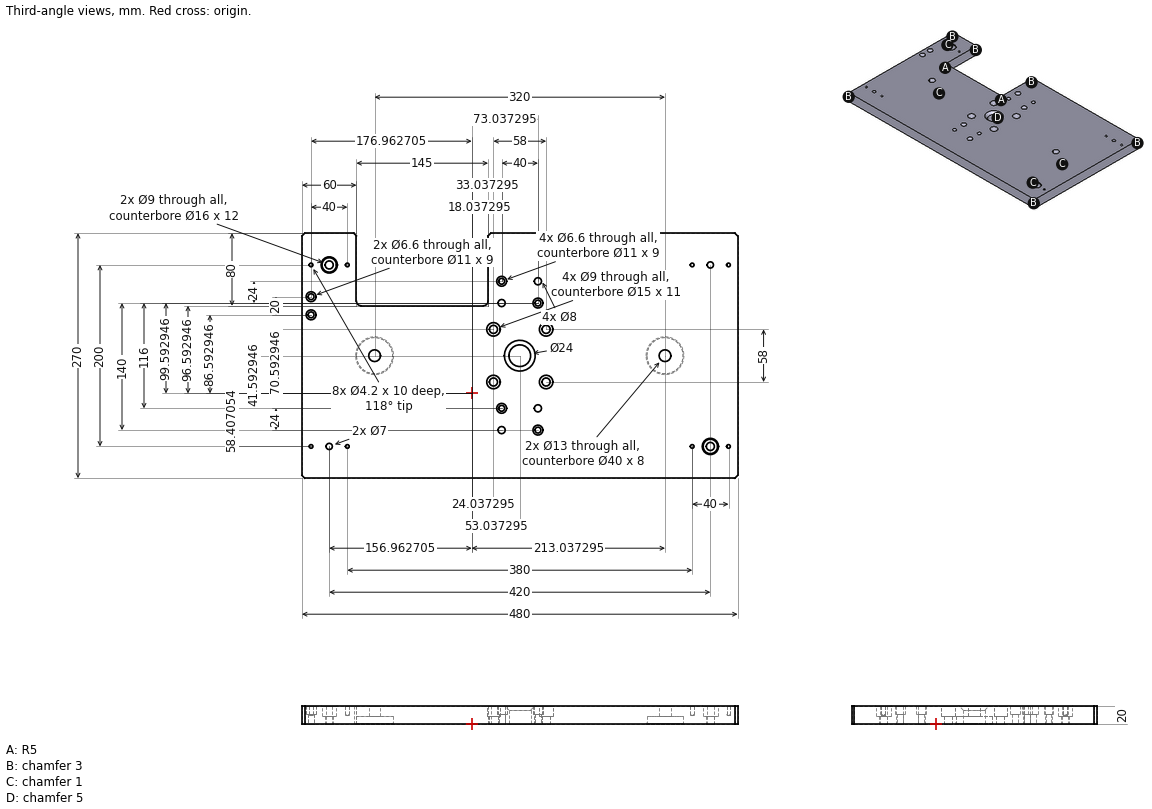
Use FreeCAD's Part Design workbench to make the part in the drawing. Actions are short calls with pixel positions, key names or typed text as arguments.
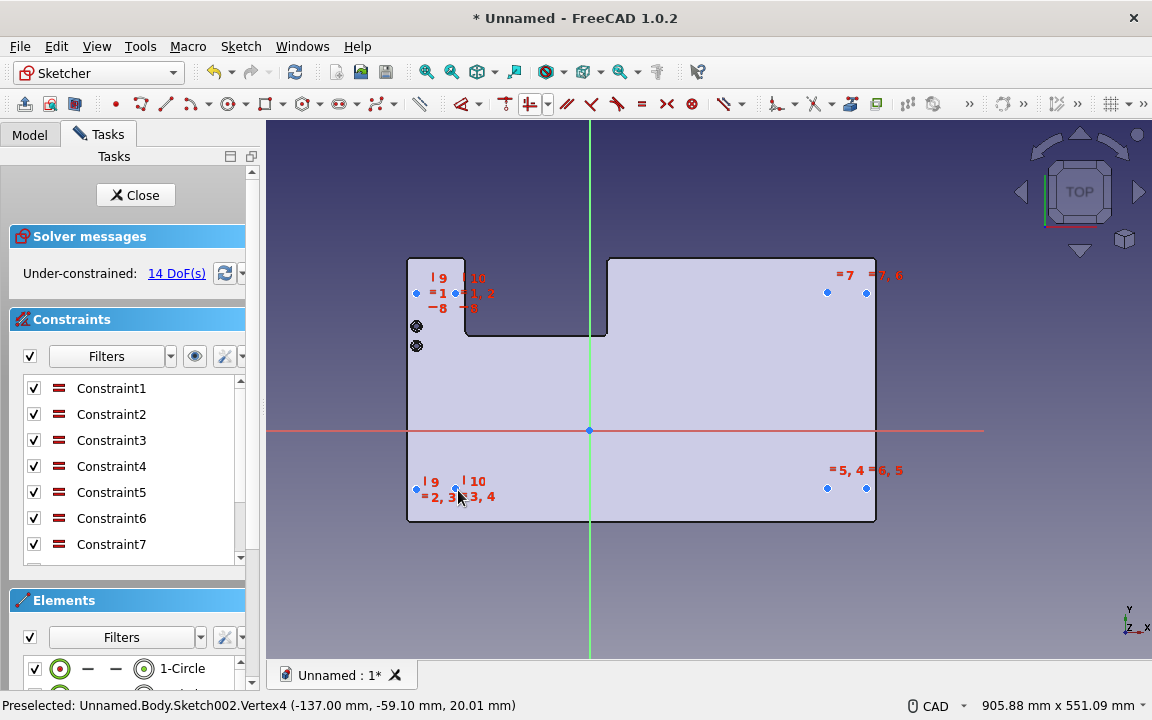
click(416, 489)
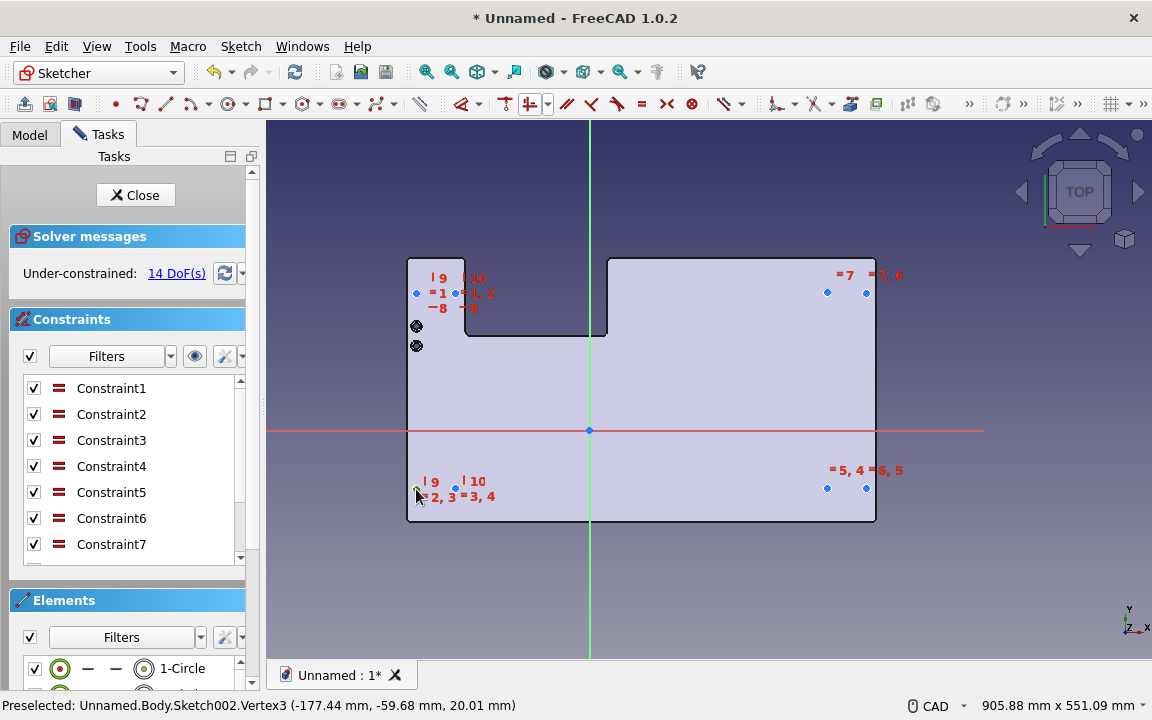
click(457, 490)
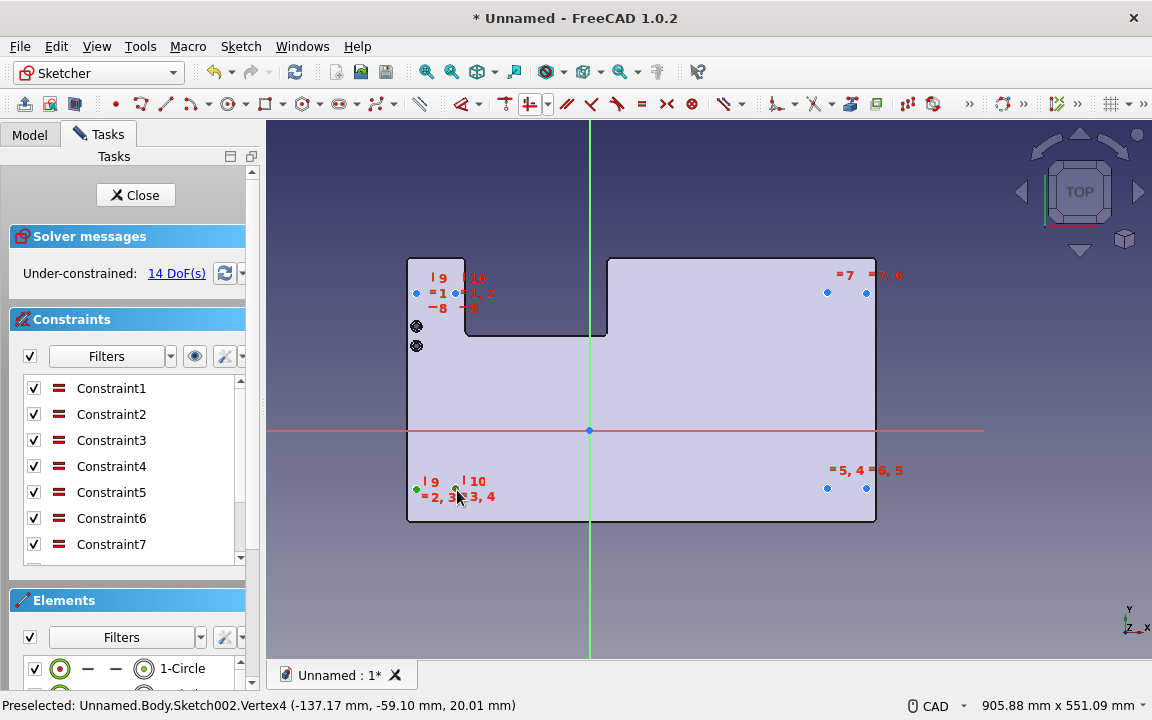
key(h)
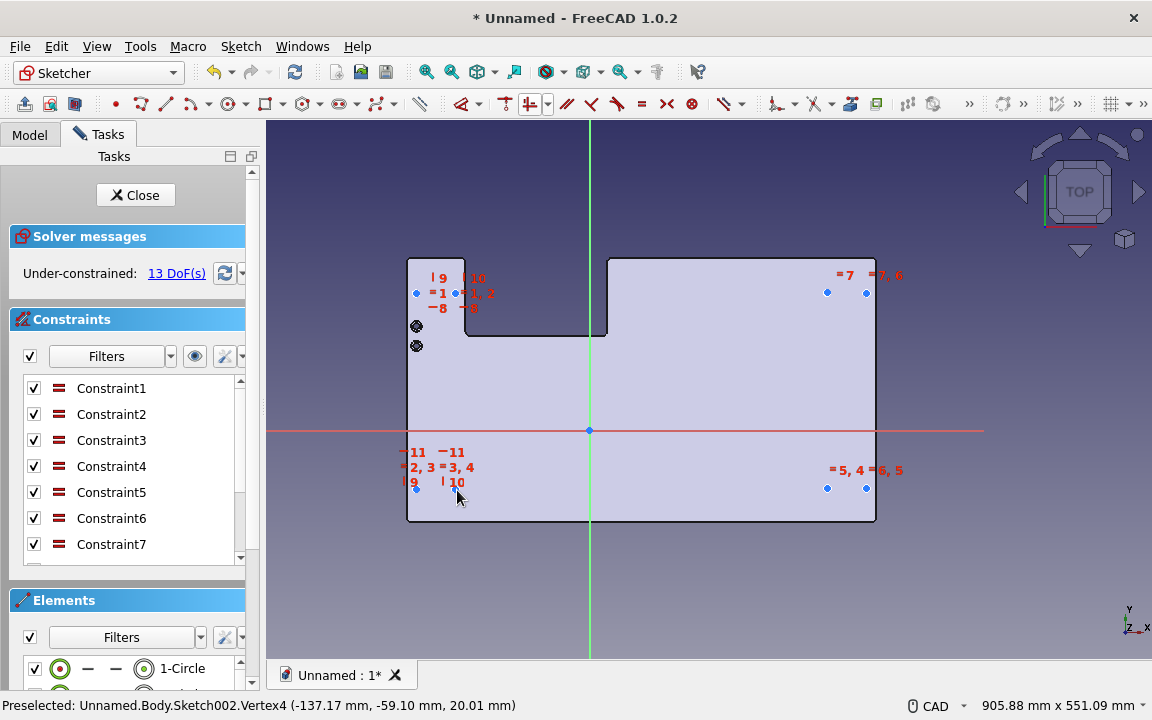
click(455, 489)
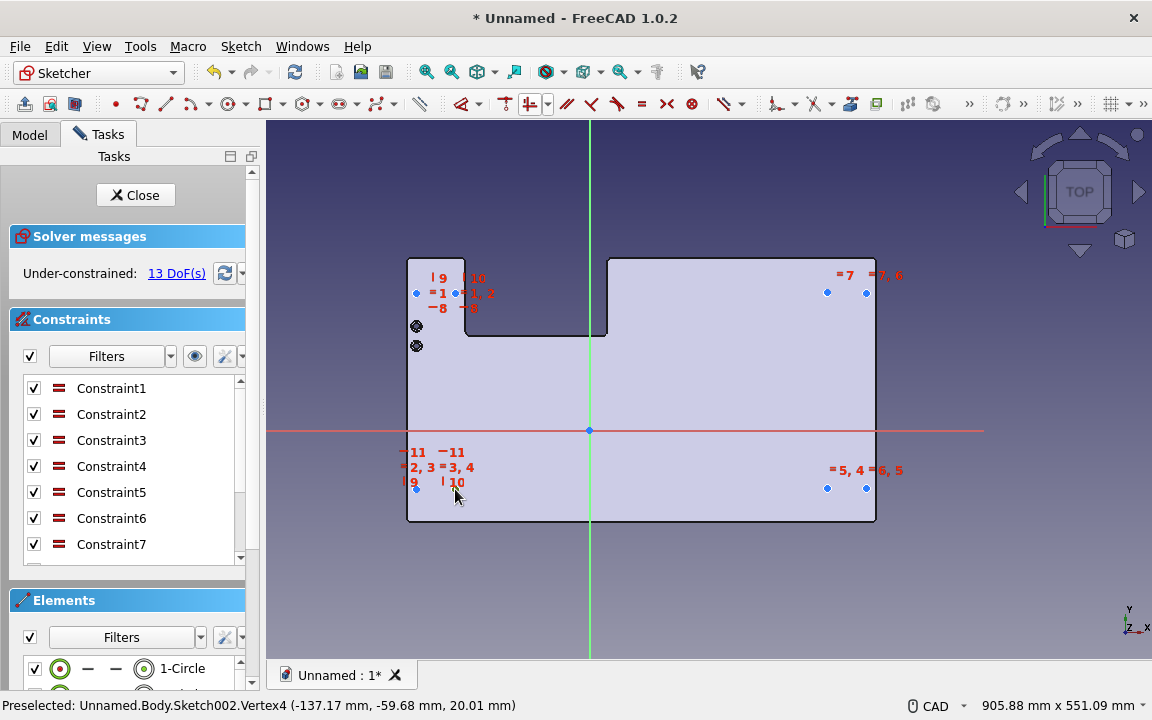
click(828, 488)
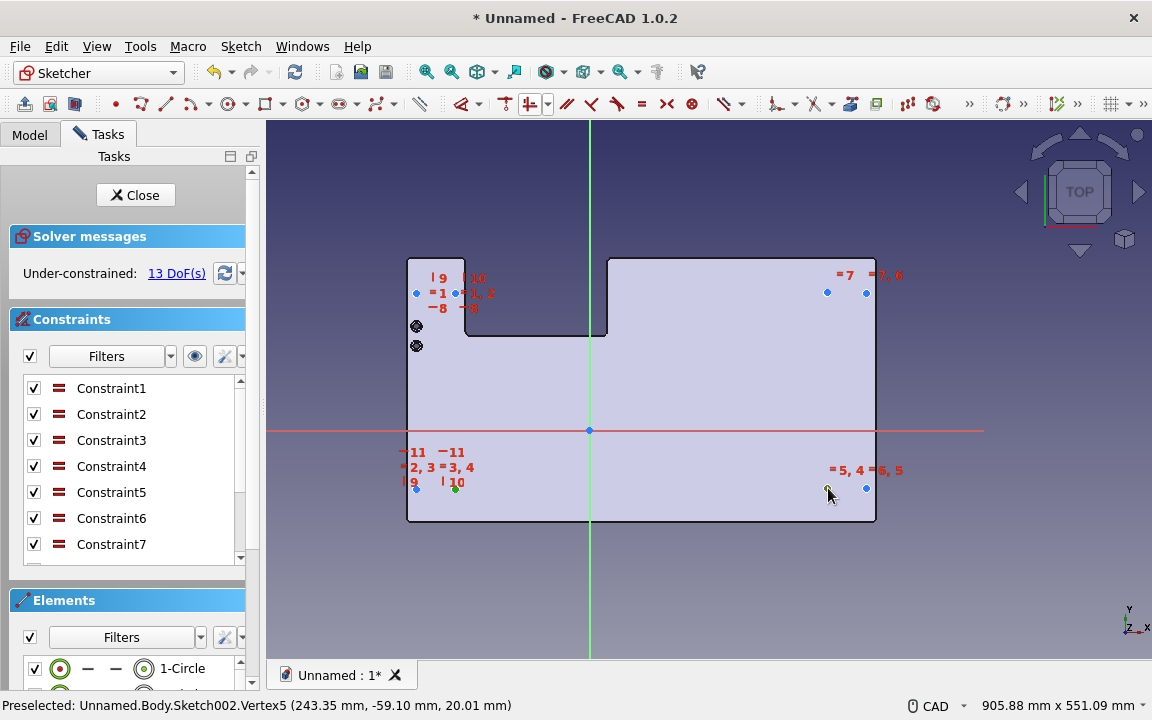
key(h)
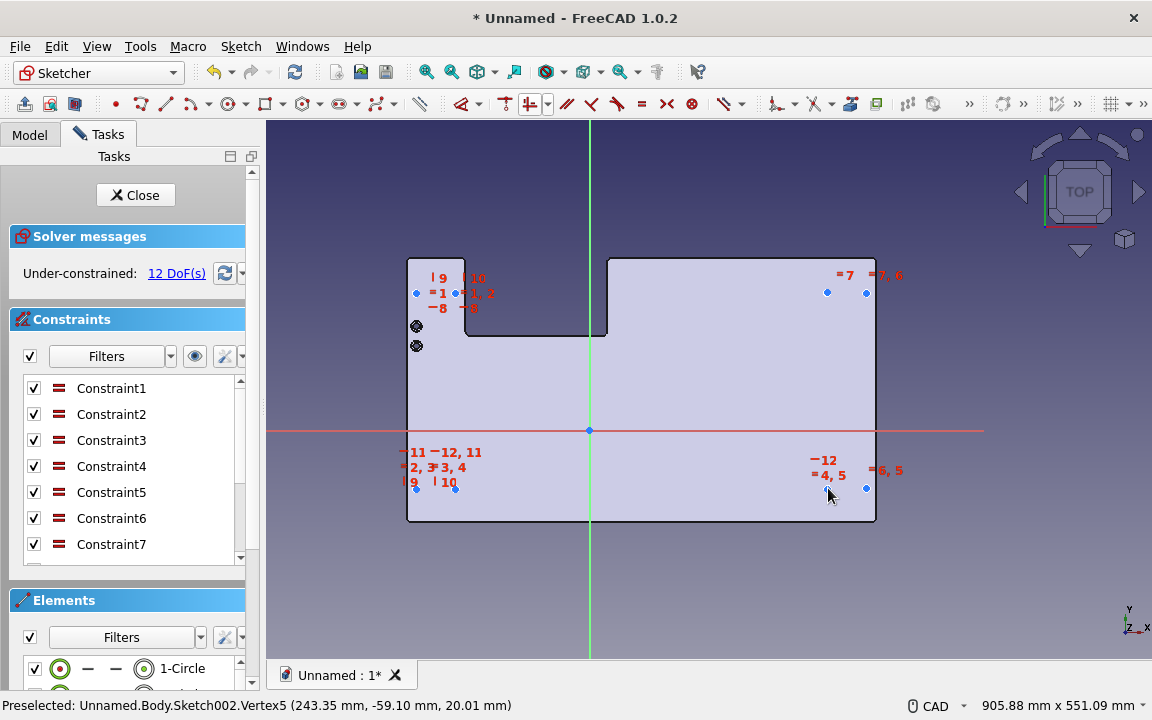
click(828, 489)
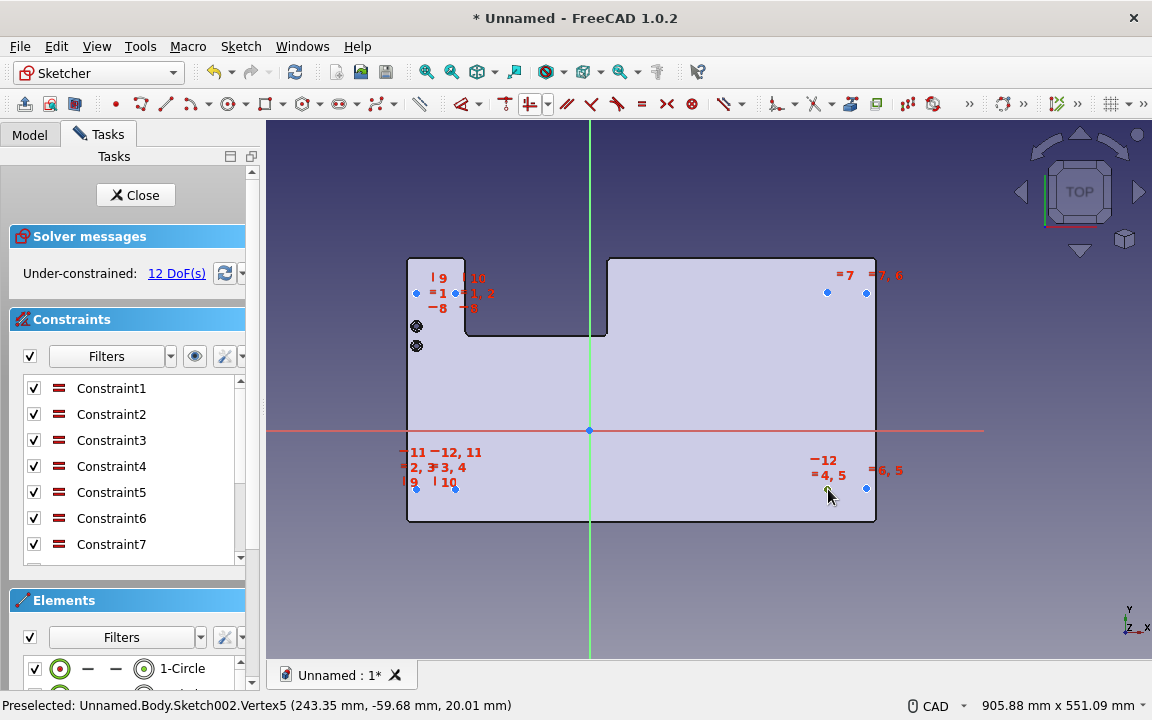
click(867, 488)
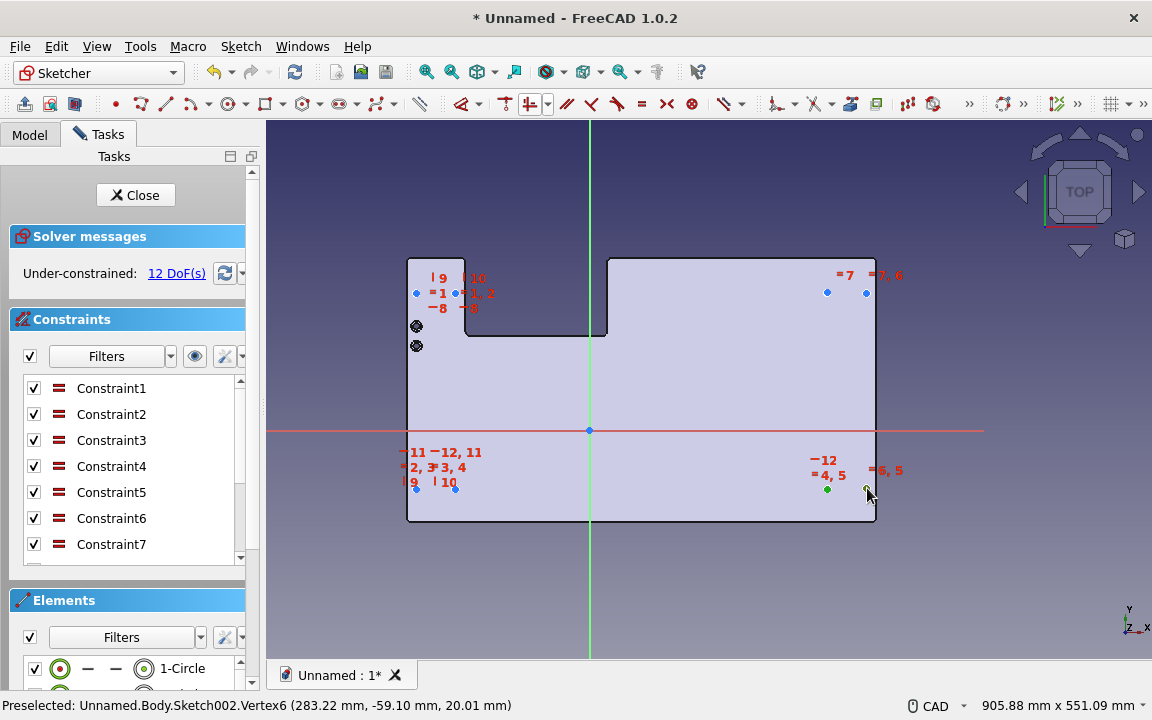
key(h)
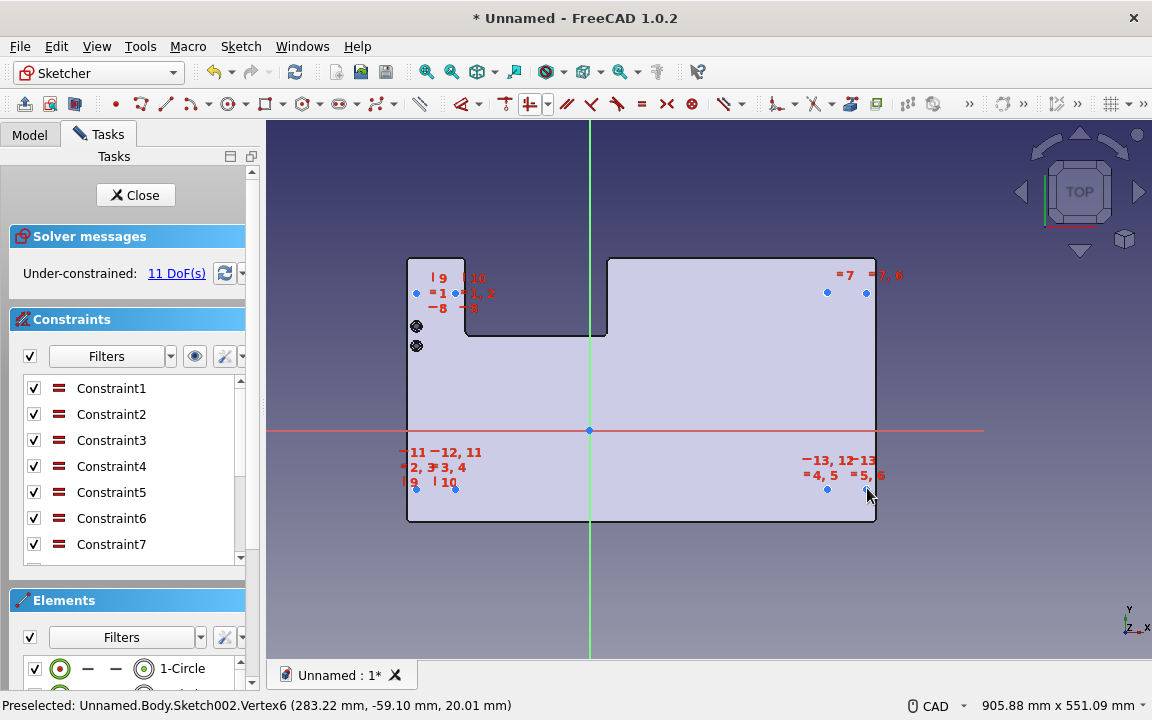
click(867, 489)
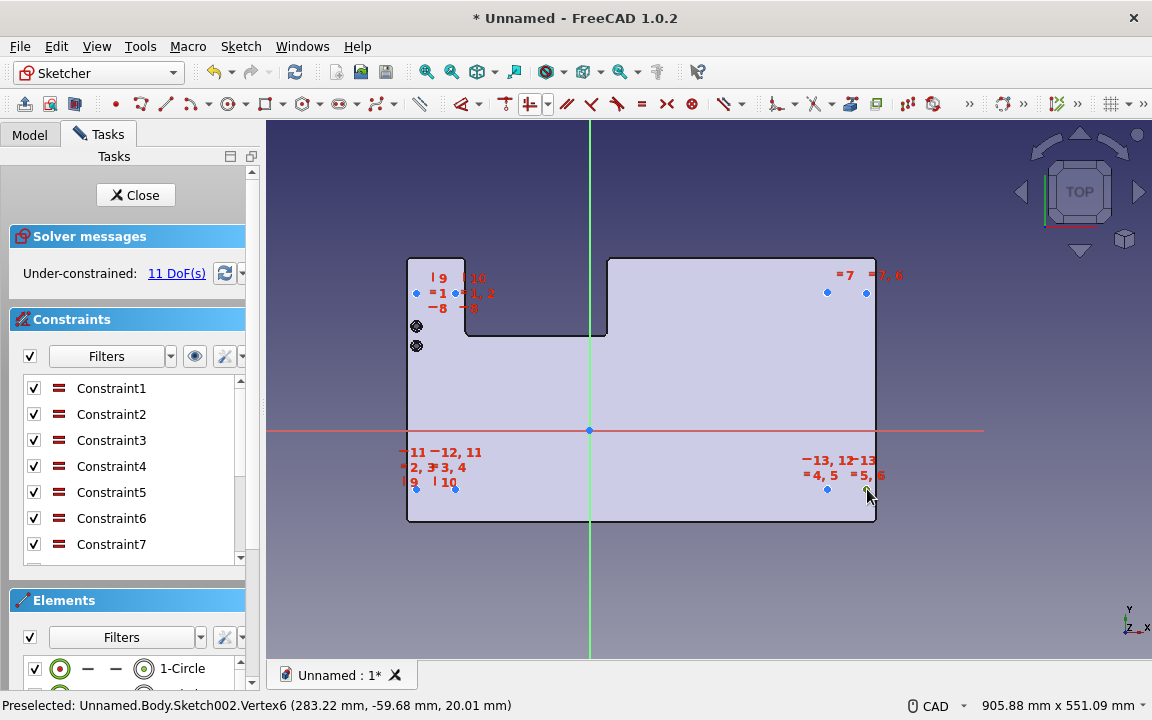
click(867, 293)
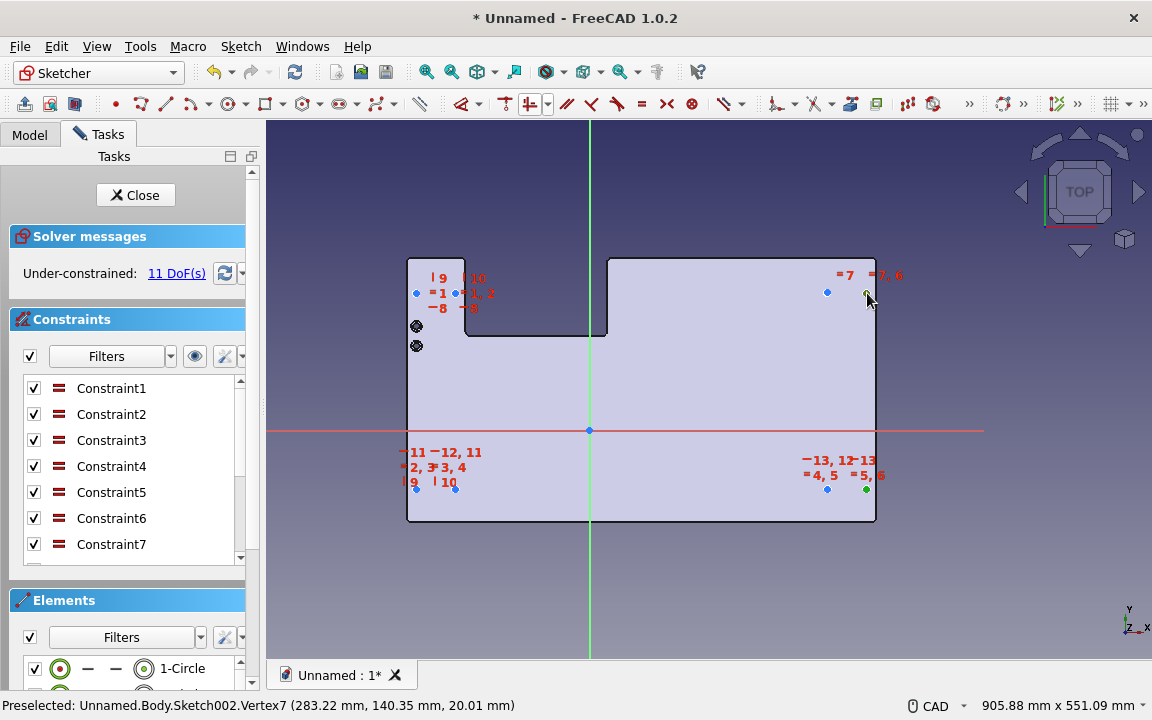
key(v)